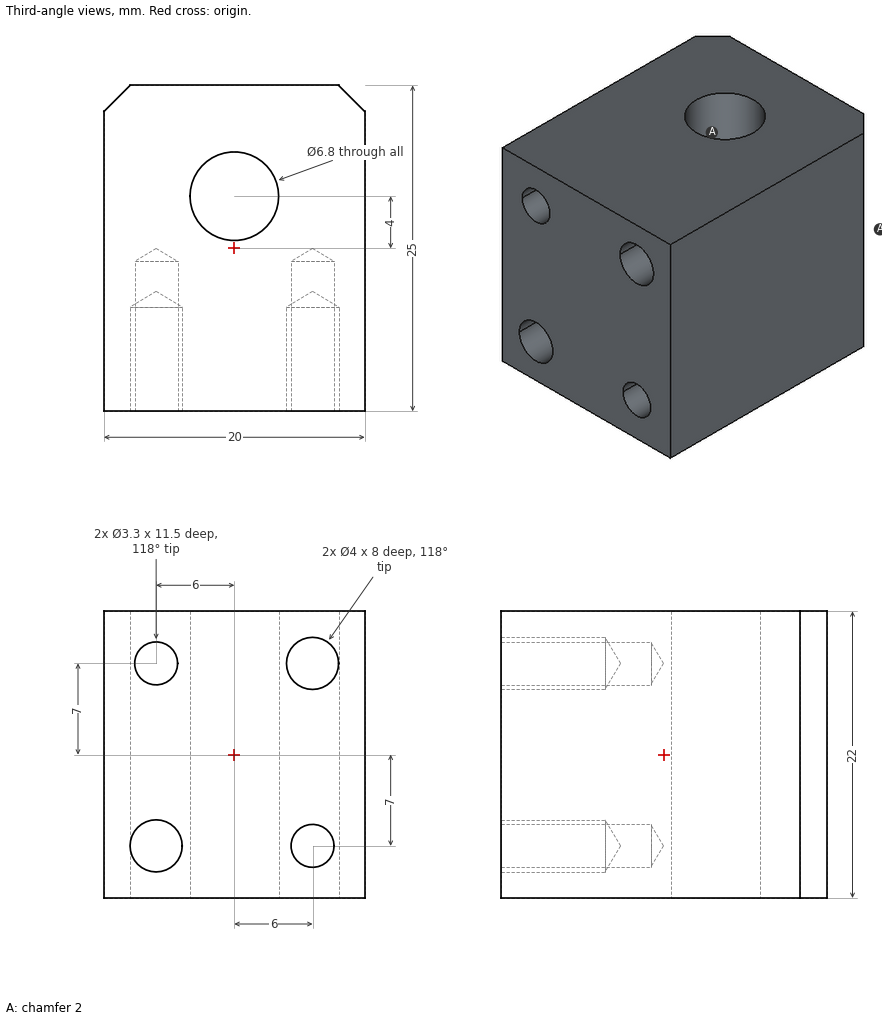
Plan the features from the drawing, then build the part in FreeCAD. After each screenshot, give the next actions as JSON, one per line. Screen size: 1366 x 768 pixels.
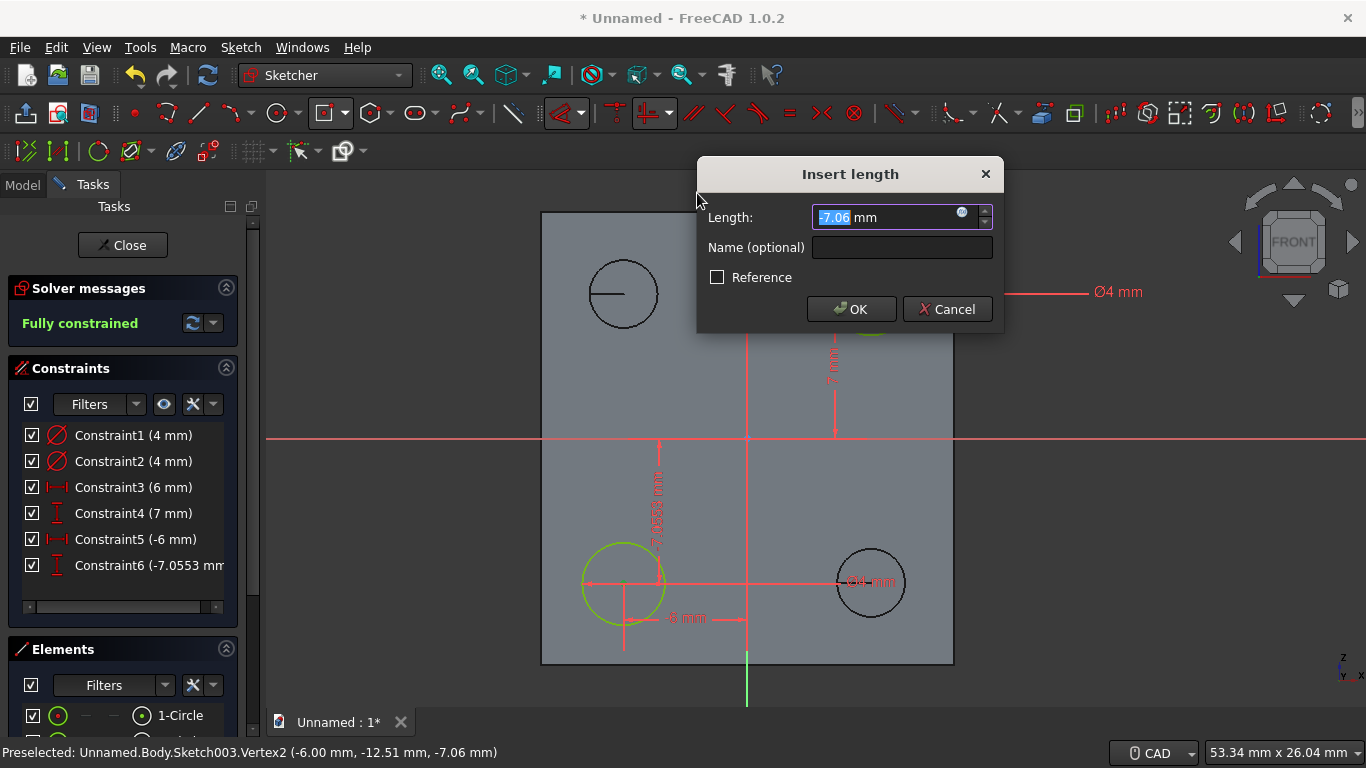
{"action": "type", "text": "-7"}
{"action": "key", "text": "Return"}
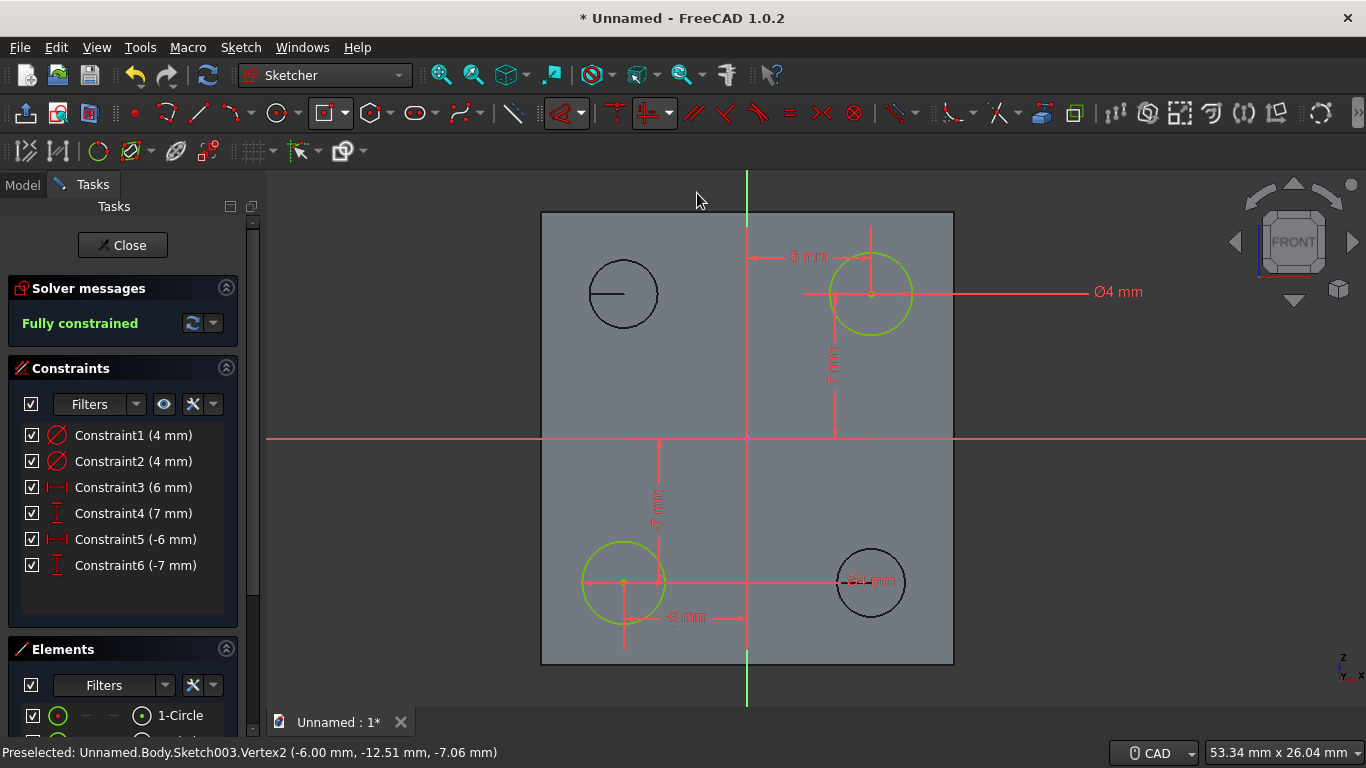
{"action": "left_click", "coordinate": [123, 245]}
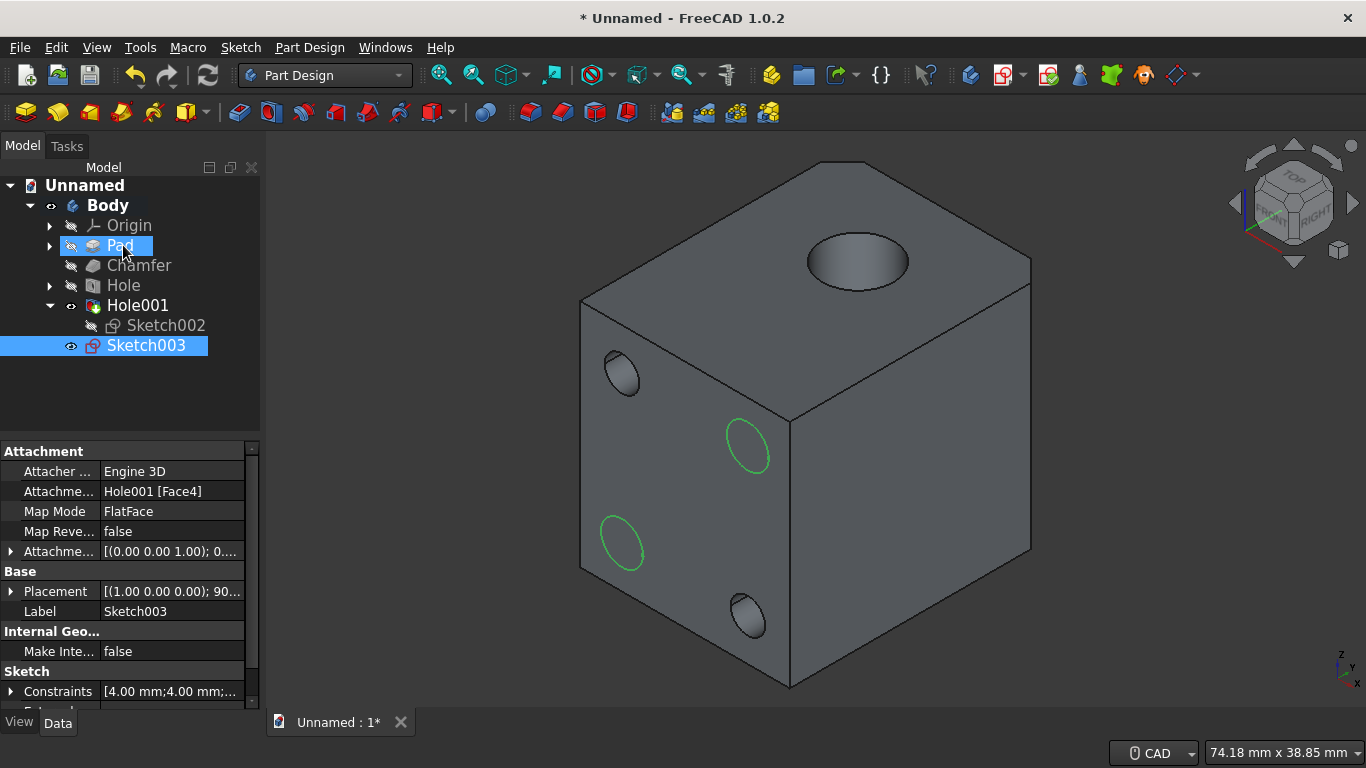
{"action": "left_click", "coordinate": [272, 112]}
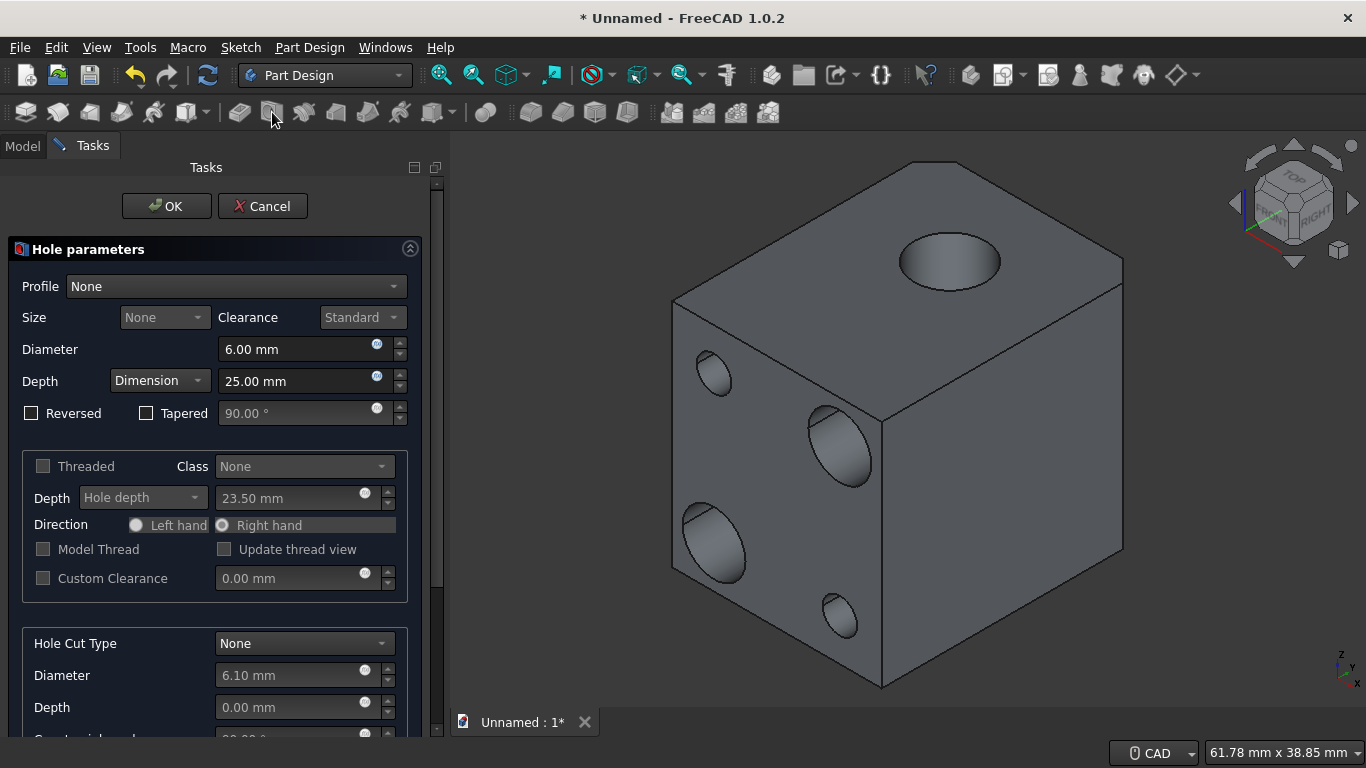
{"action": "triple_click", "coordinate": [305, 349]}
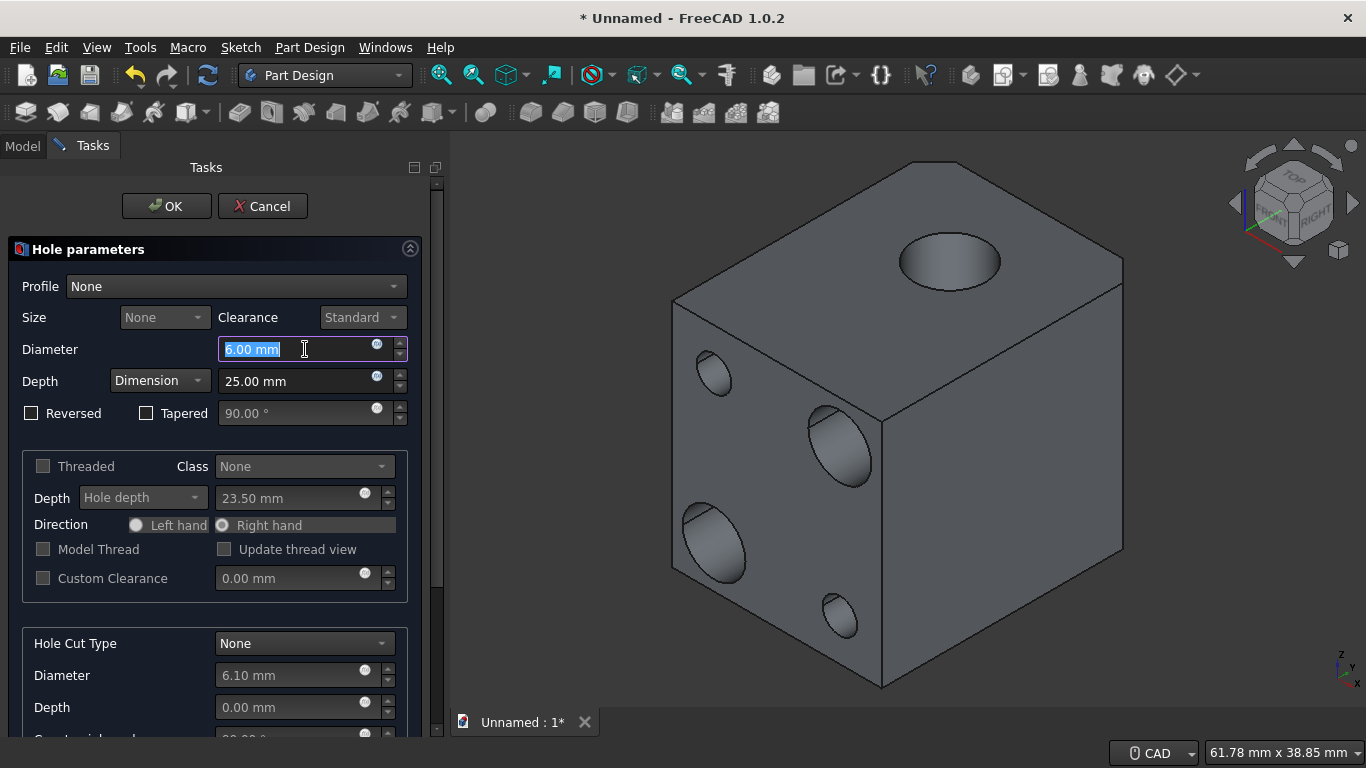
{"action": "type", "text": "4"}
{"action": "key", "text": "Tab"}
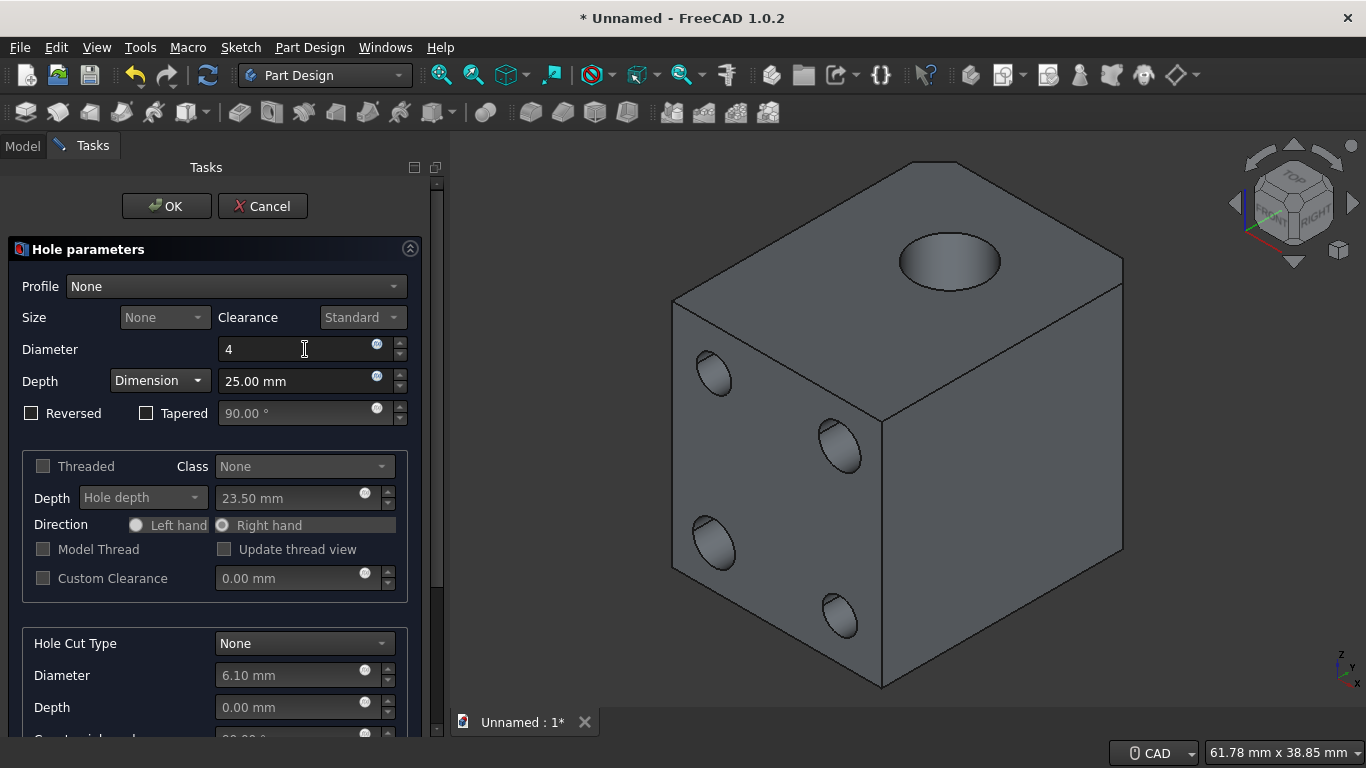
{"action": "triple_click", "coordinate": [305, 381]}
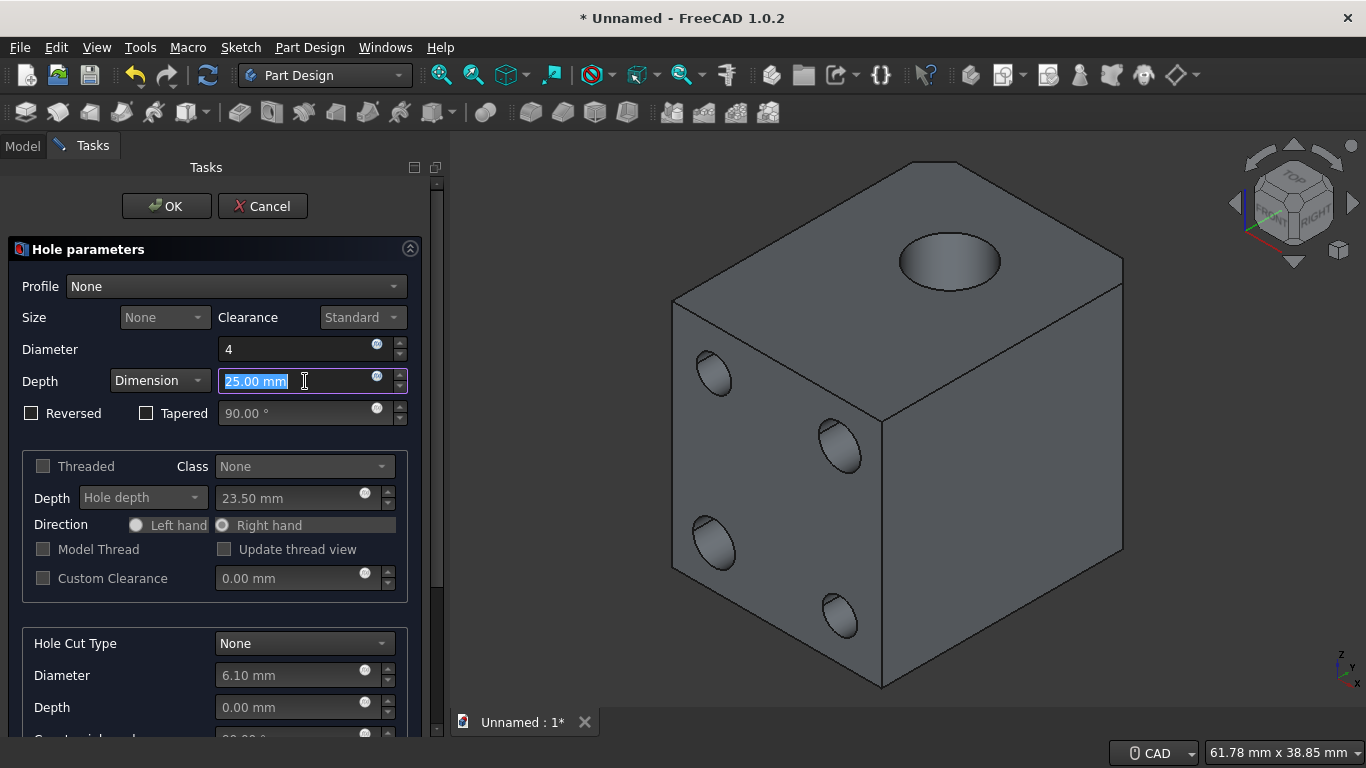
{"action": "type", "text": "8"}
{"action": "key", "text": "Tab"}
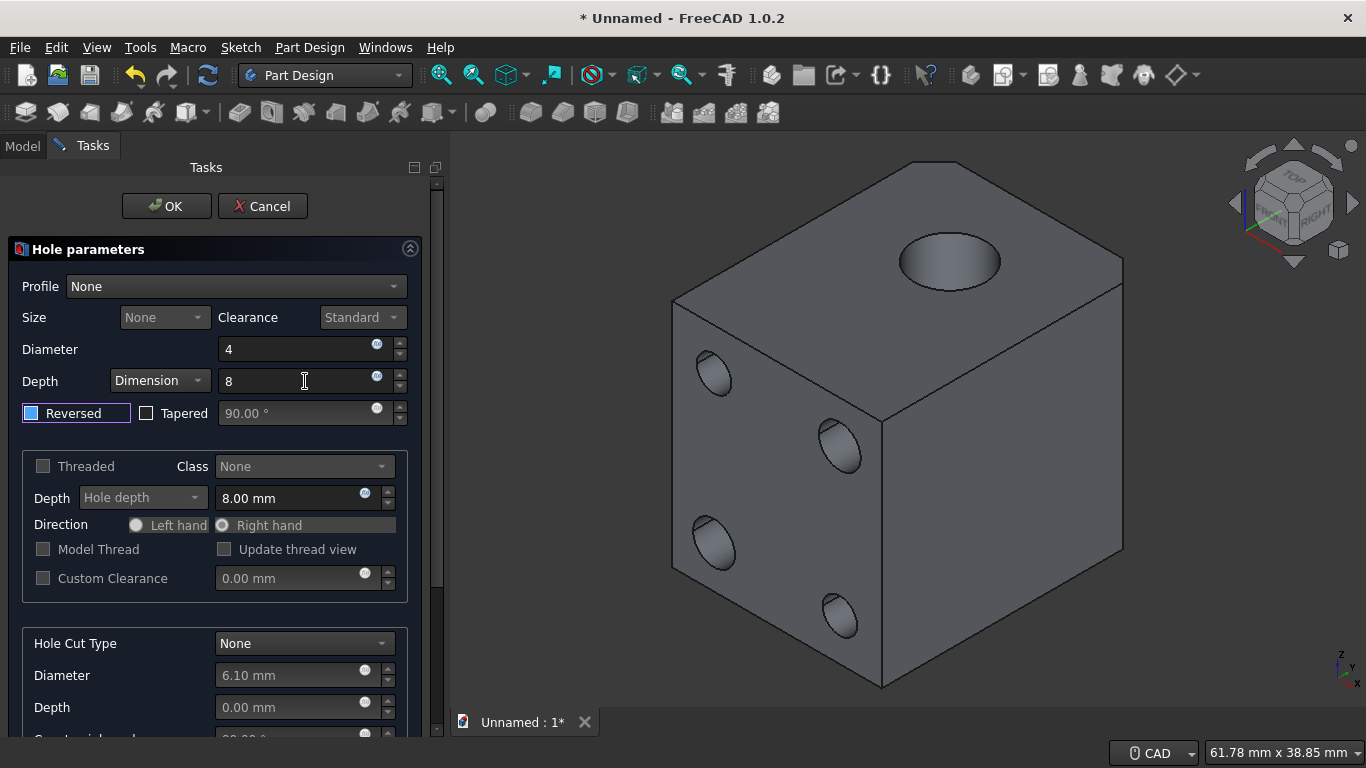
{"action": "left_click", "coordinate": [167, 206]}